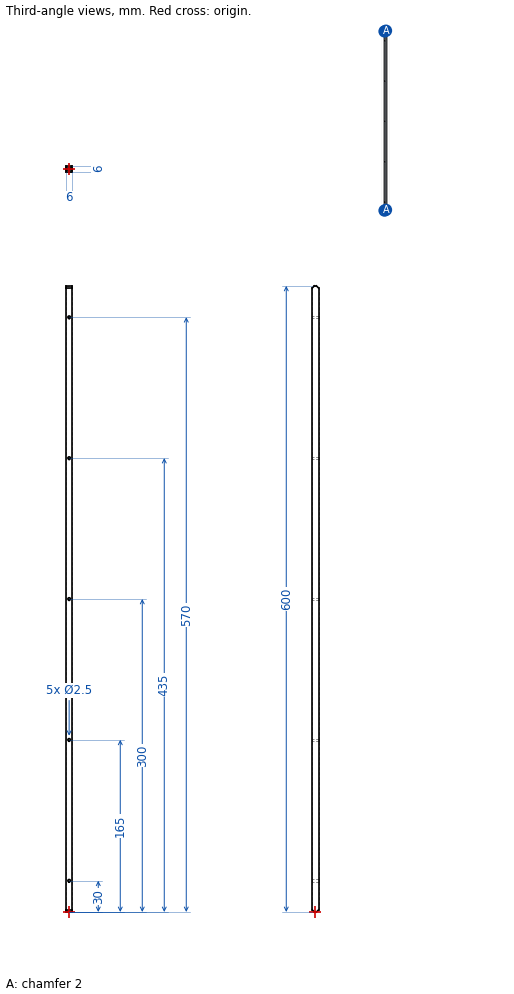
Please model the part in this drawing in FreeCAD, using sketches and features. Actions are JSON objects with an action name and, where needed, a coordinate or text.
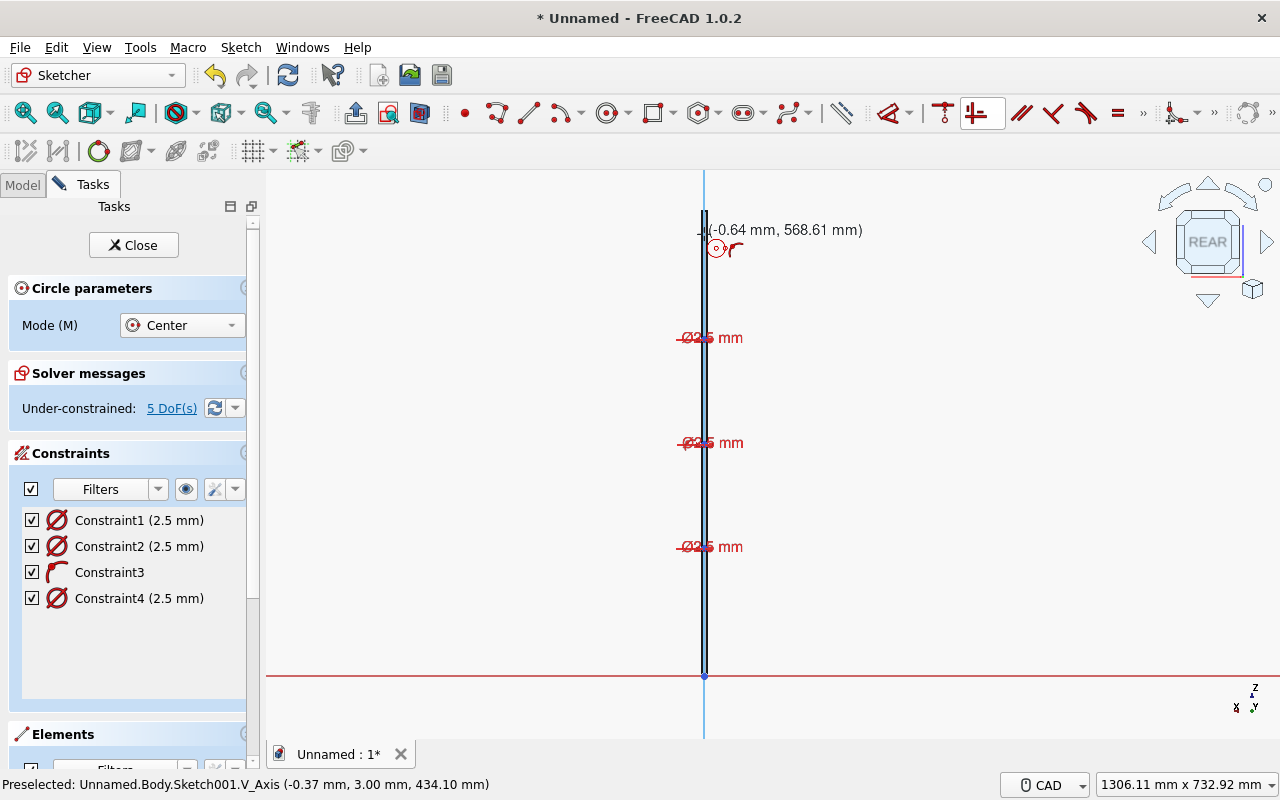
{"action": "left_click", "coordinate": [704, 234]}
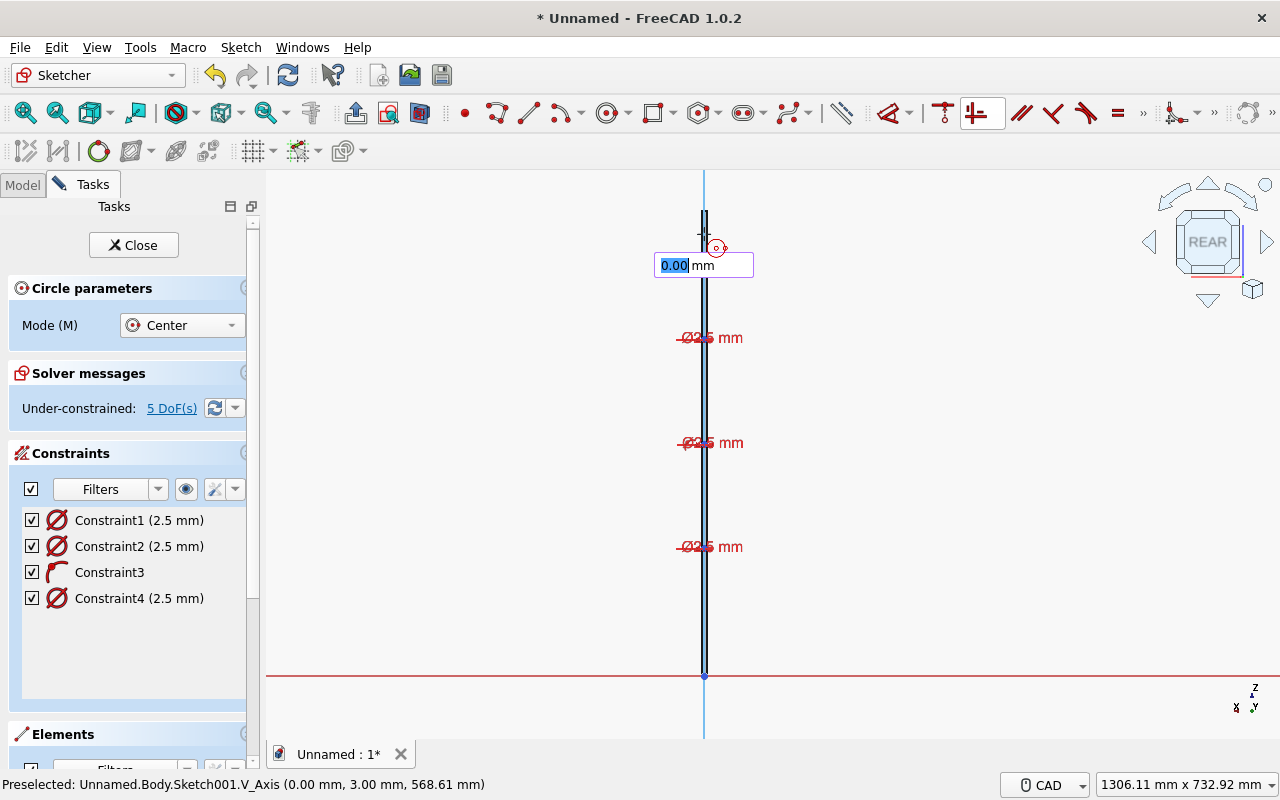
{"action": "scroll", "coordinate": [705, 234], "scroll_direction": "up", "scroll_amount": 15}
{"action": "mouse_move", "coordinate": [705, 224]}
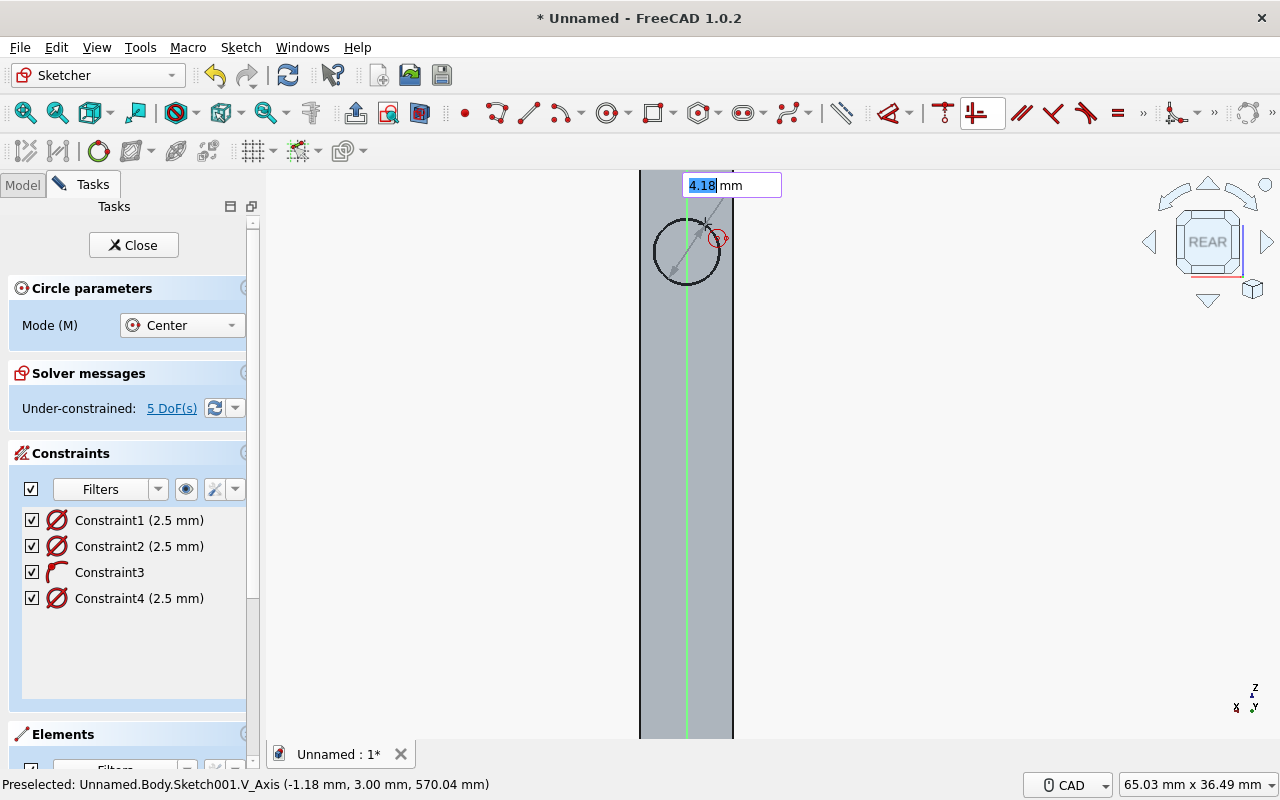
{"action": "type", "text": "2.5"}
{"action": "key", "text": "Return"}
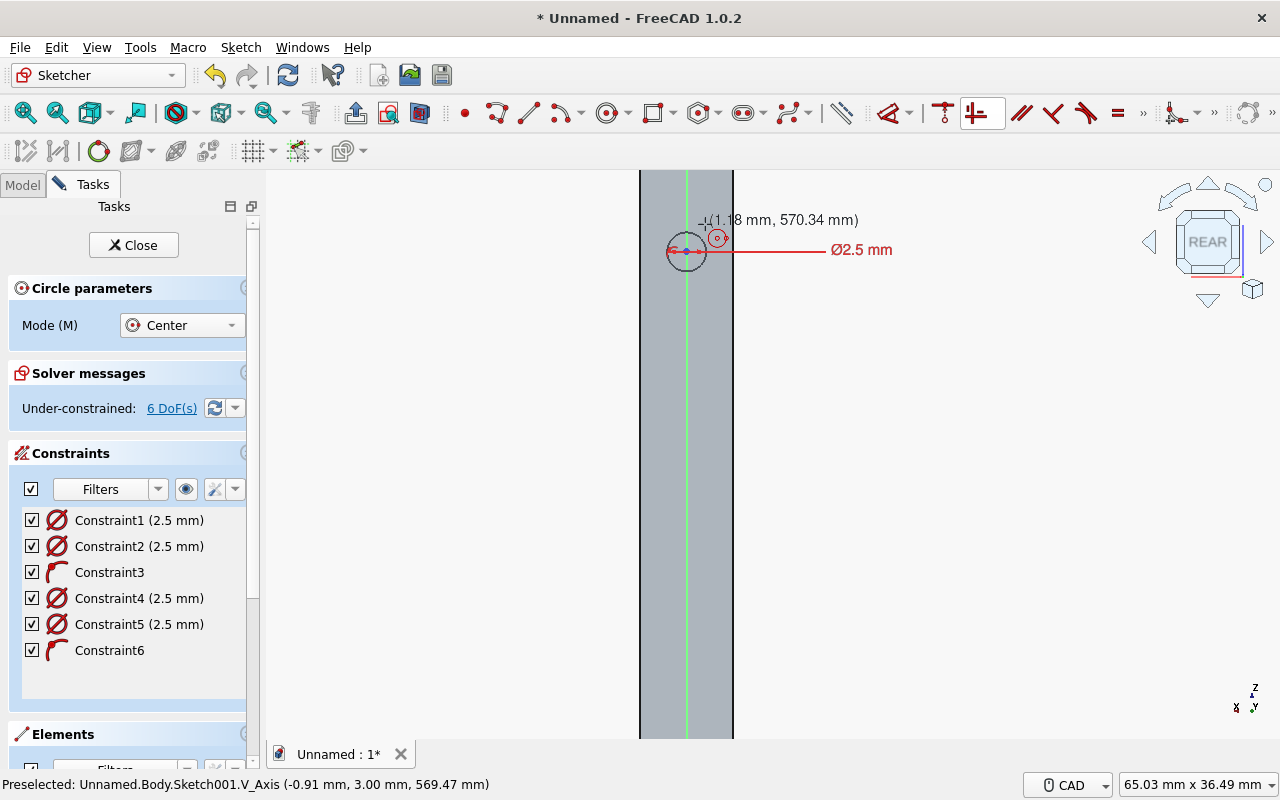
{"action": "scroll", "coordinate": [705, 234], "scroll_direction": "down", "scroll_amount": 15}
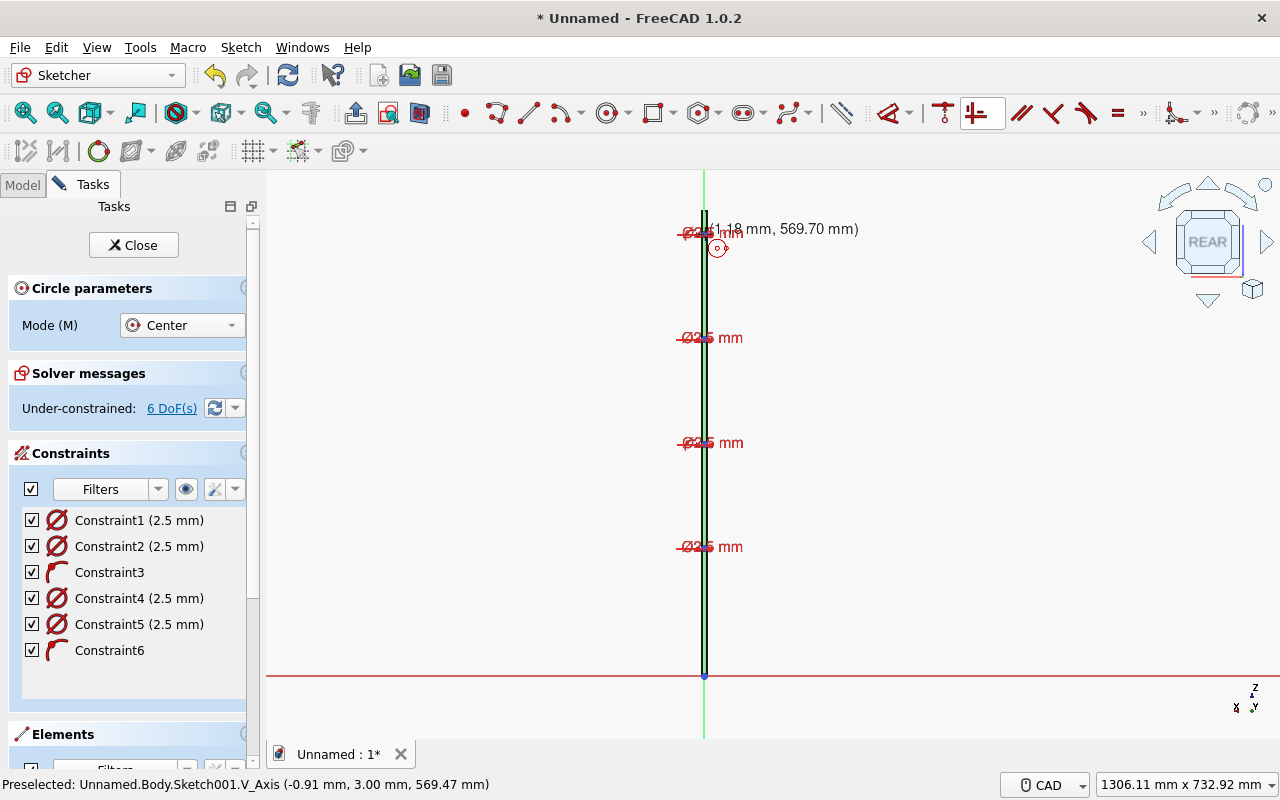
{"action": "scroll", "coordinate": [704, 653], "scroll_direction": "up", "scroll_amount": 16}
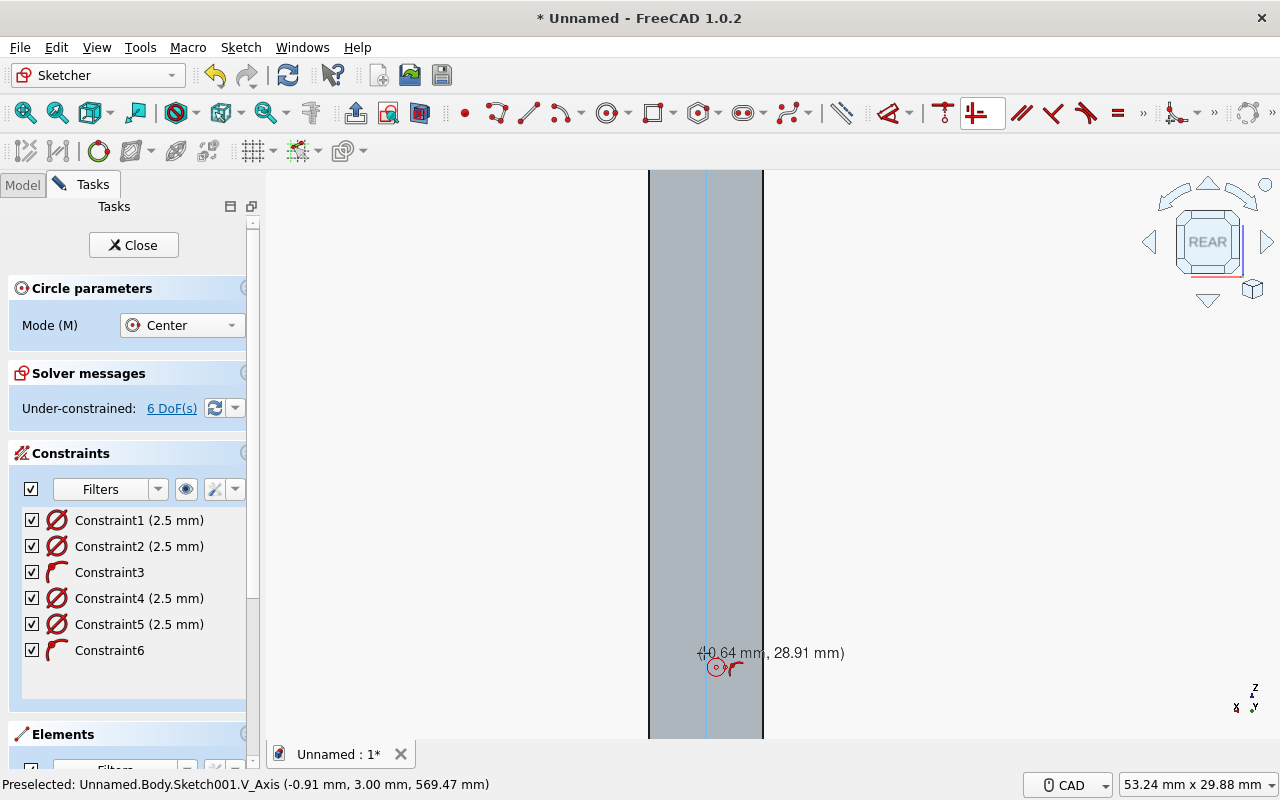
{"action": "scroll", "coordinate": [704, 654], "scroll_direction": "down", "scroll_amount": 16}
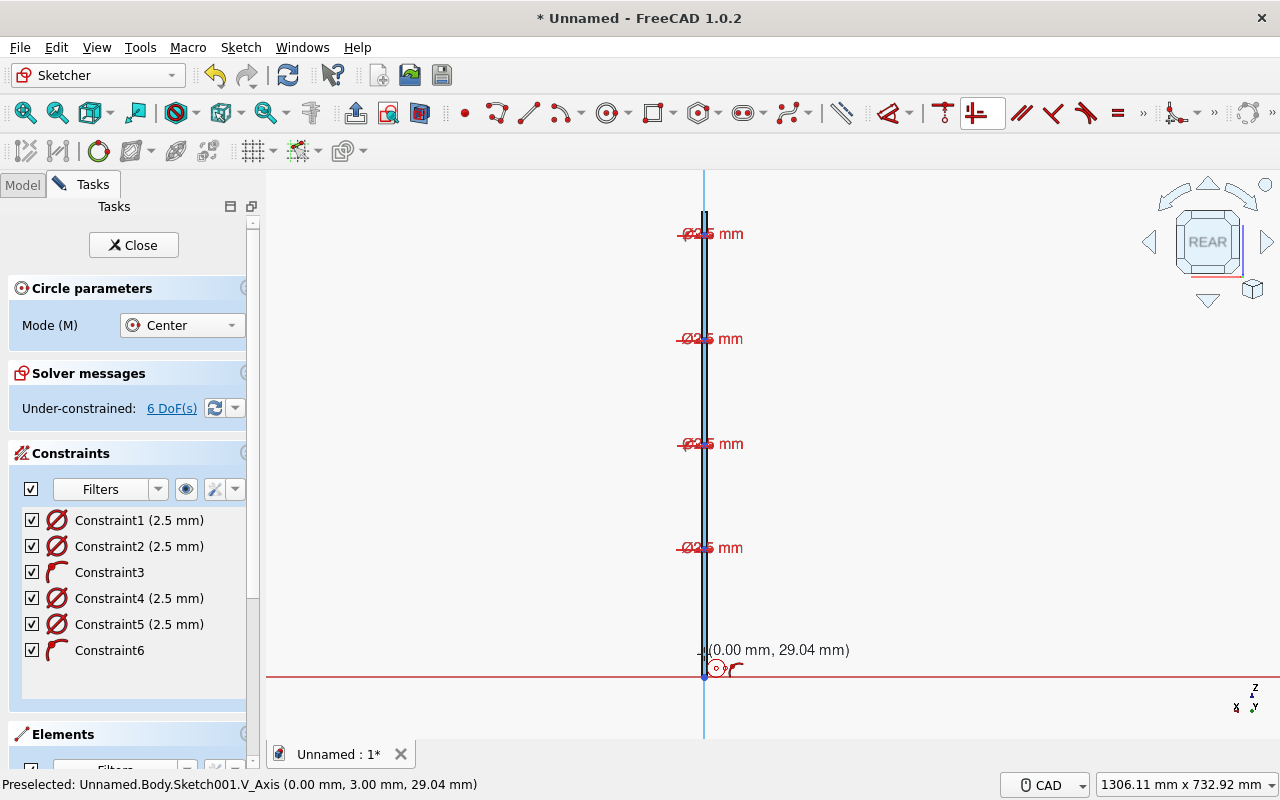
{"action": "left_click", "coordinate": [704, 654]}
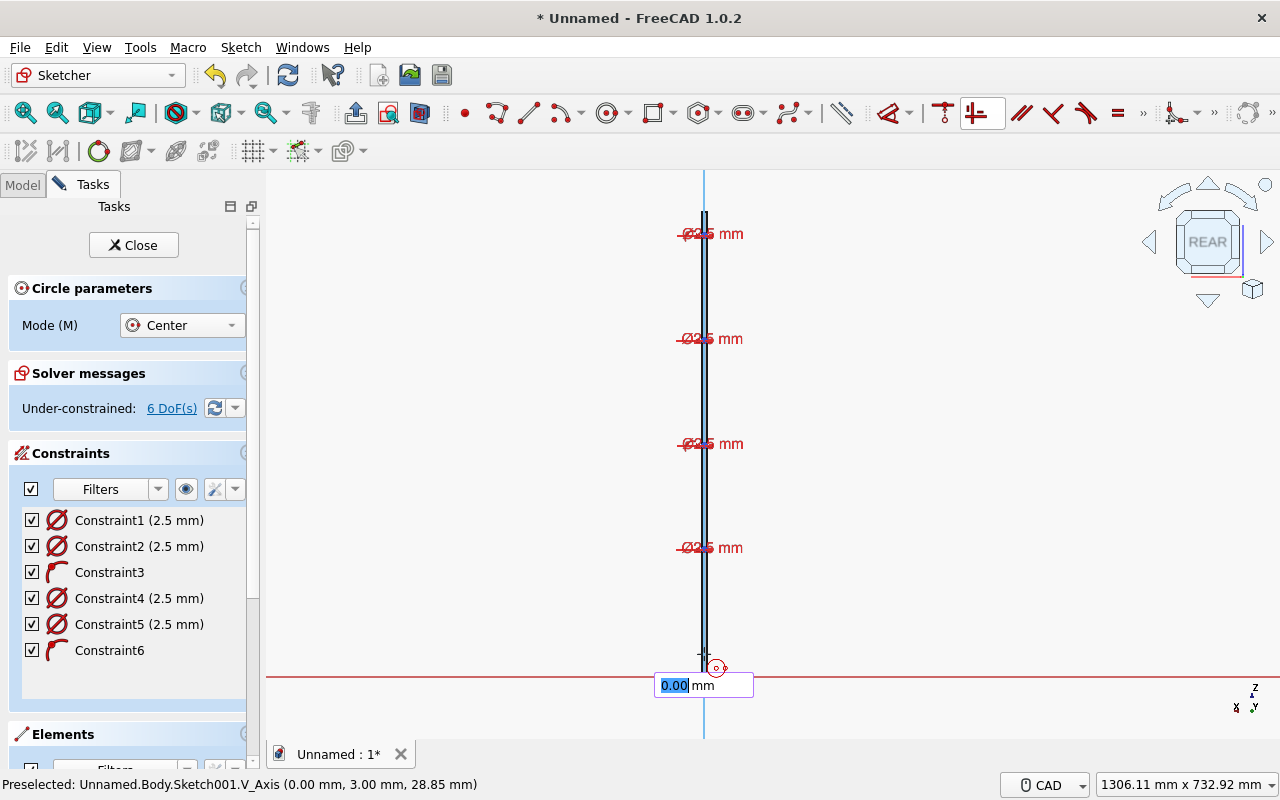
{"action": "scroll", "coordinate": [705, 654], "scroll_direction": "up", "scroll_amount": 15}
{"action": "mouse_move", "coordinate": [705, 633]}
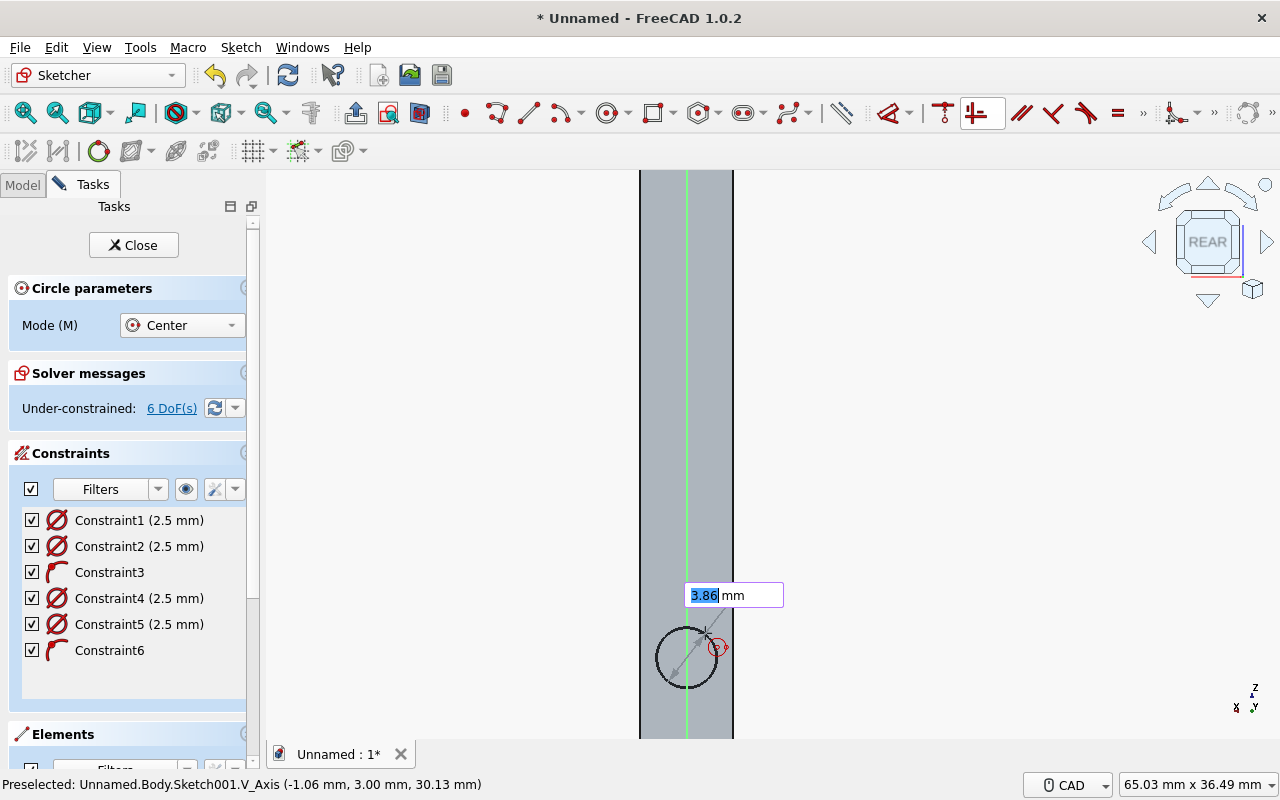
{"action": "type", "text": "2.5"}
{"action": "key", "text": "Return"}
{"action": "key", "text": "Escape"}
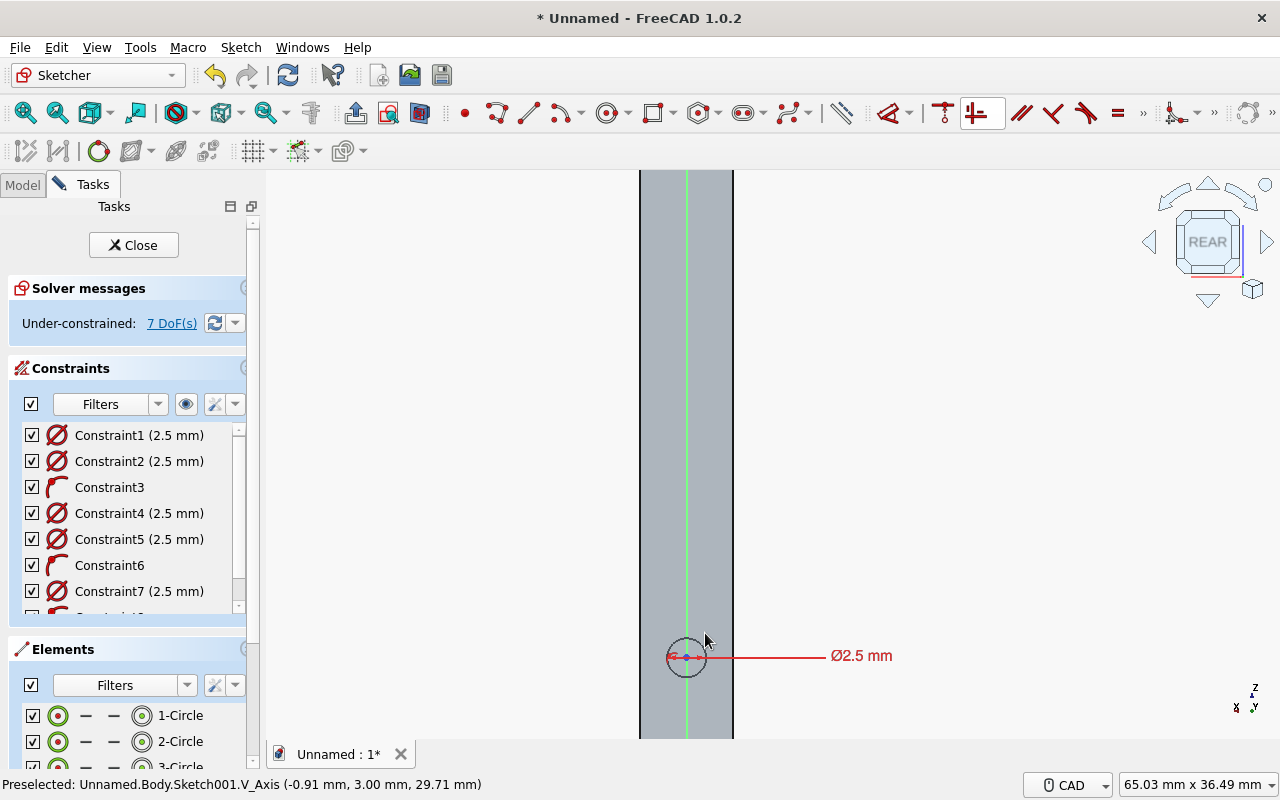
{"action": "scroll", "coordinate": [705, 654], "scroll_direction": "down", "scroll_amount": 15}